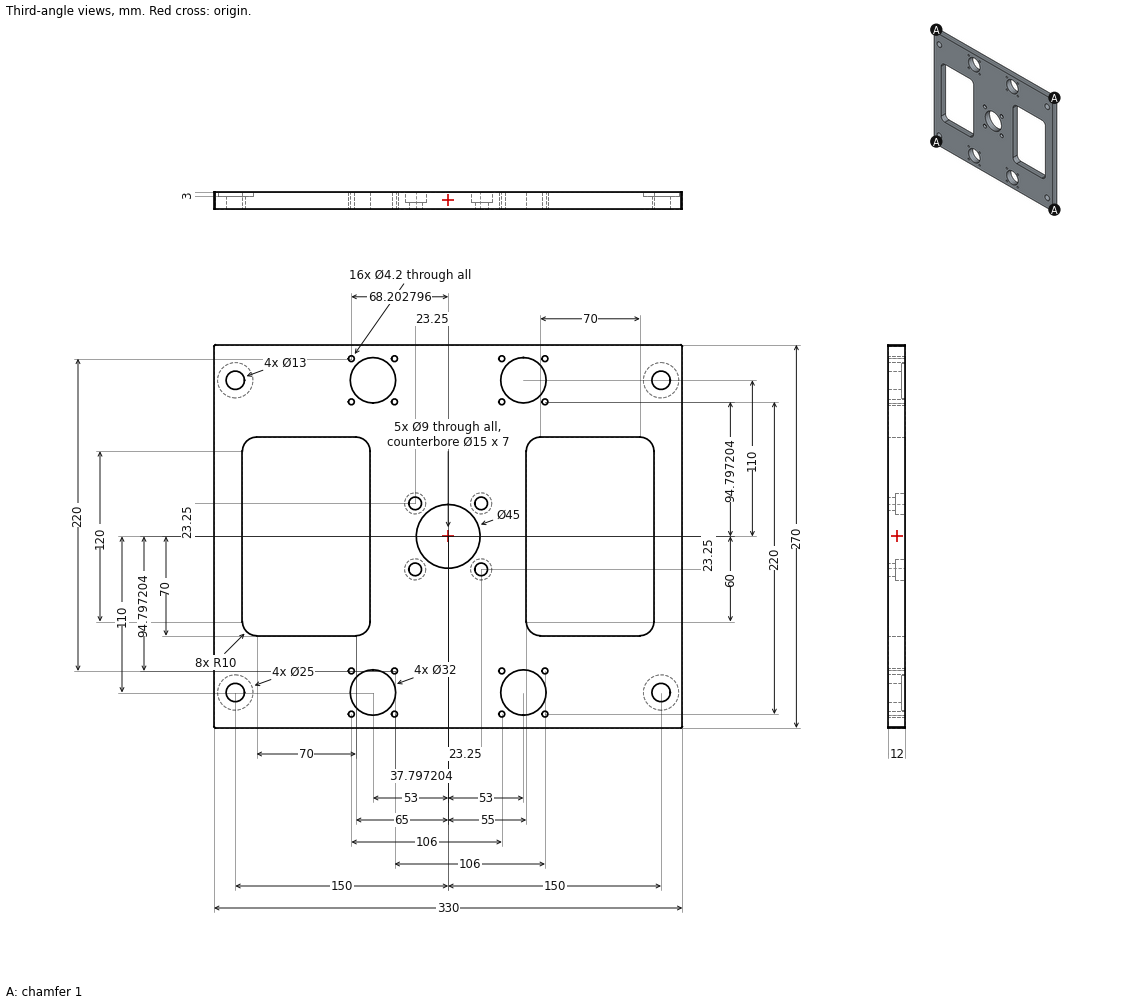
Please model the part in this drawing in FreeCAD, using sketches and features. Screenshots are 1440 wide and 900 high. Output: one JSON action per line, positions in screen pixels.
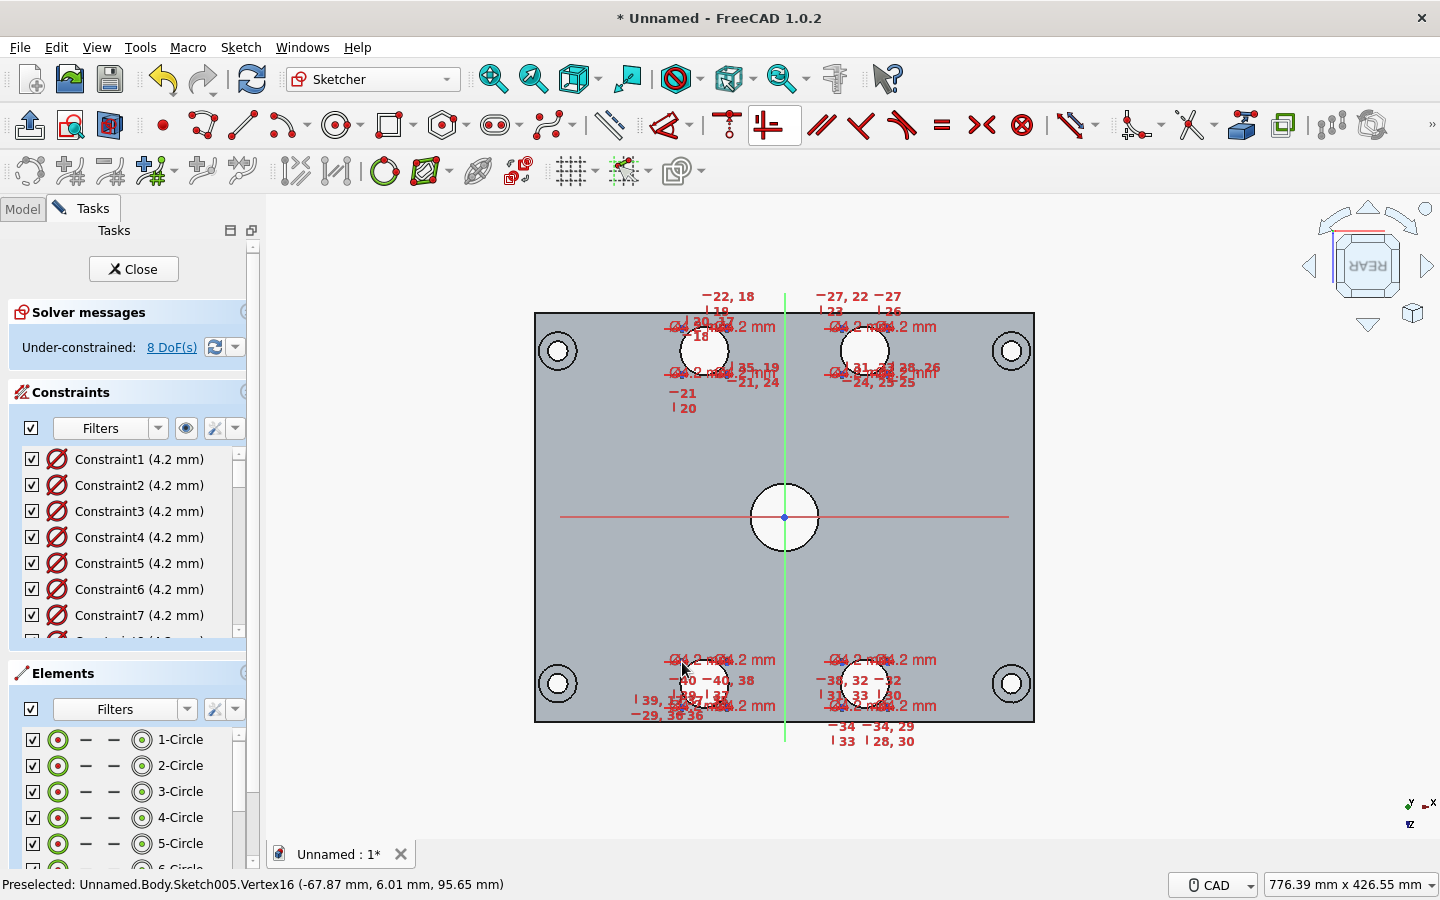
{"action": "left_click", "coordinate": [664, 126]}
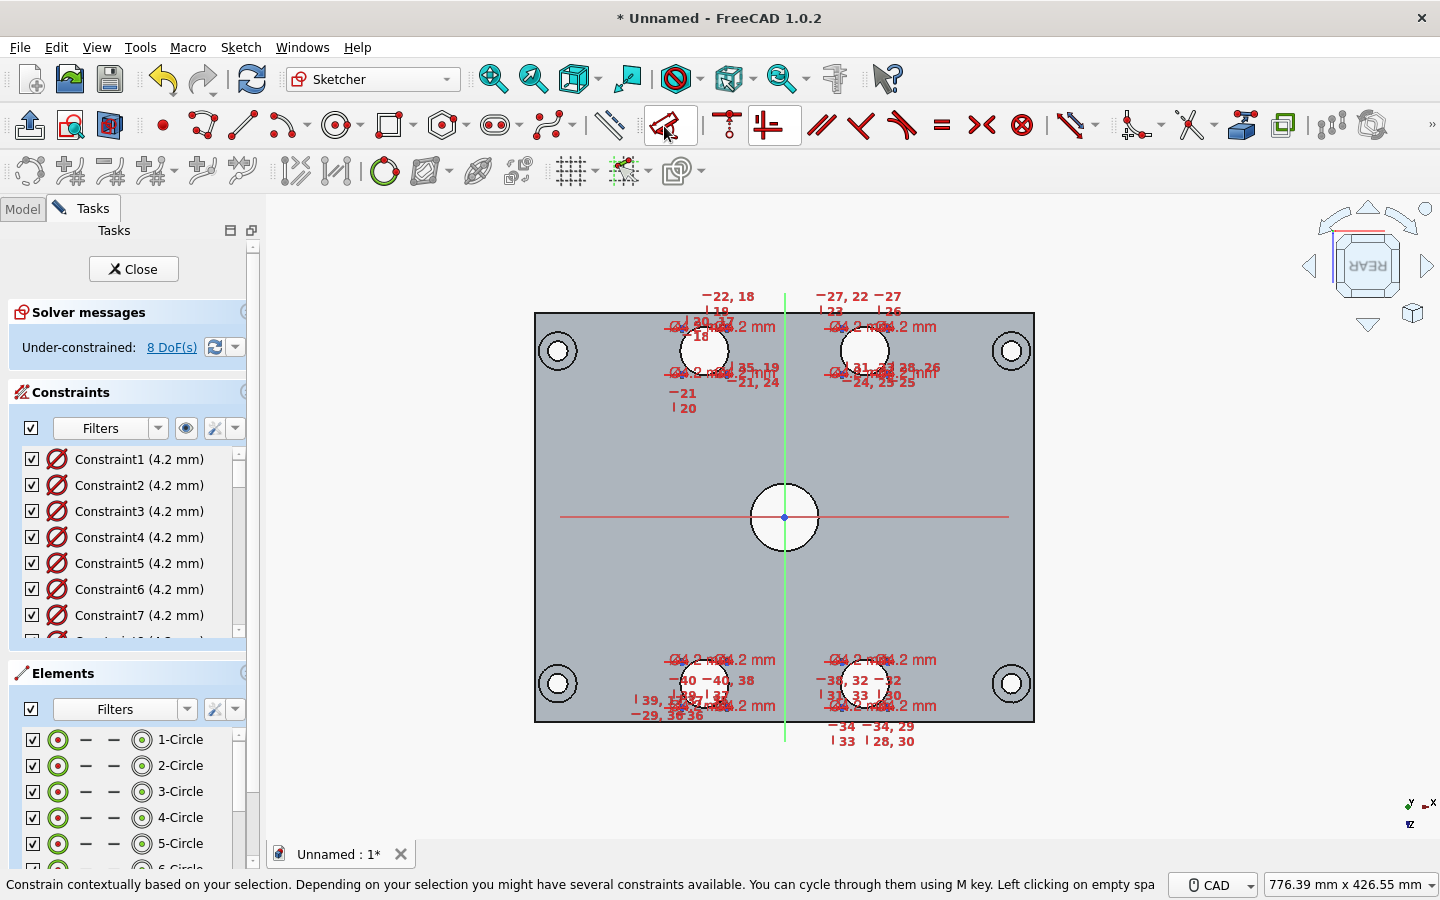
{"action": "left_click", "coordinate": [682, 708]}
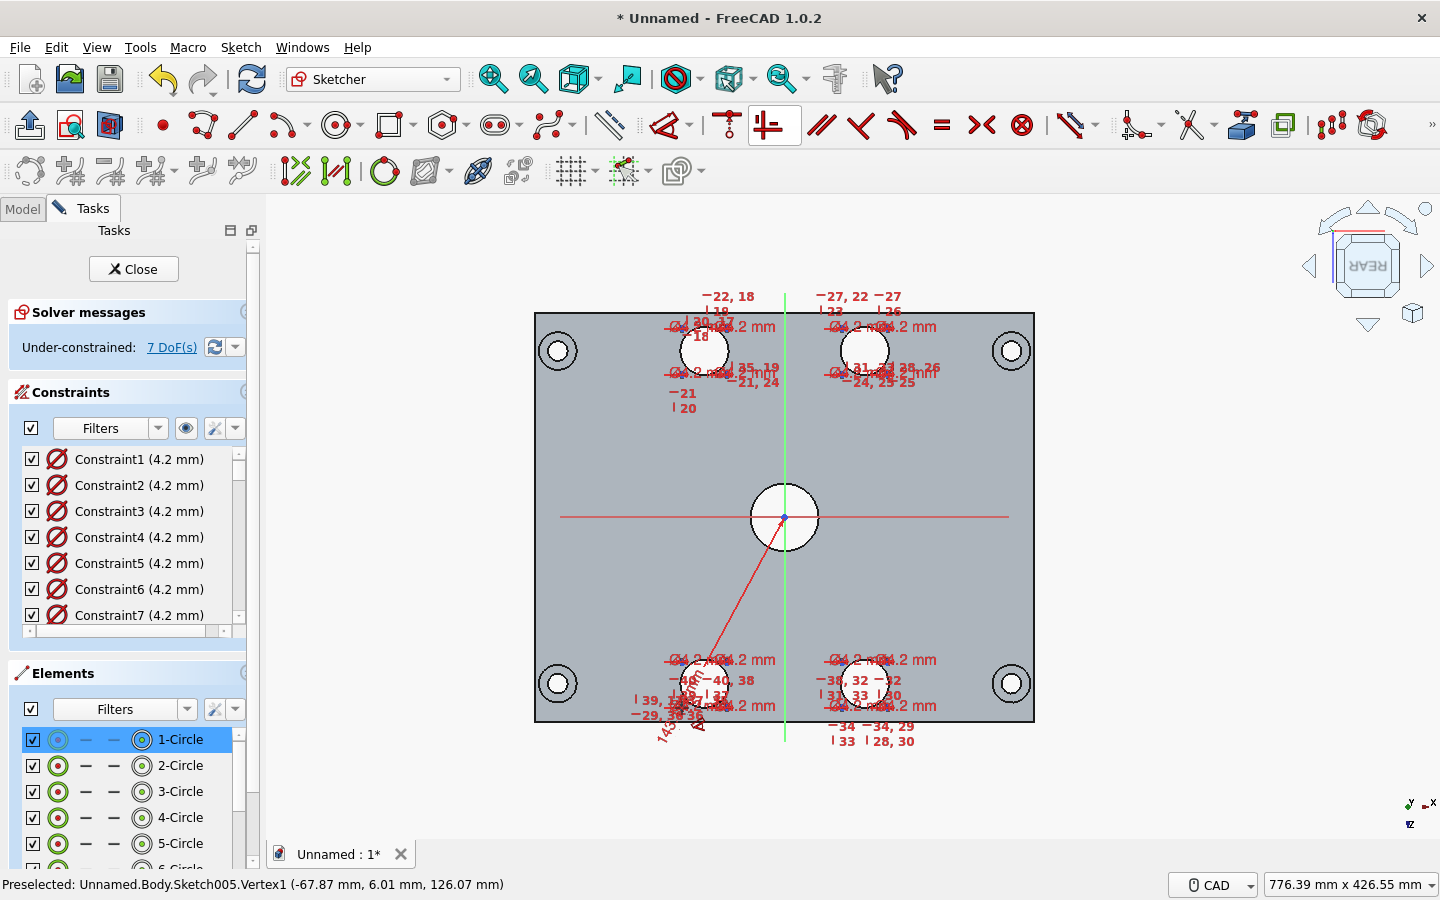
{"action": "left_click", "coordinate": [727, 375]}
{"action": "left_click", "coordinate": [648, 541]}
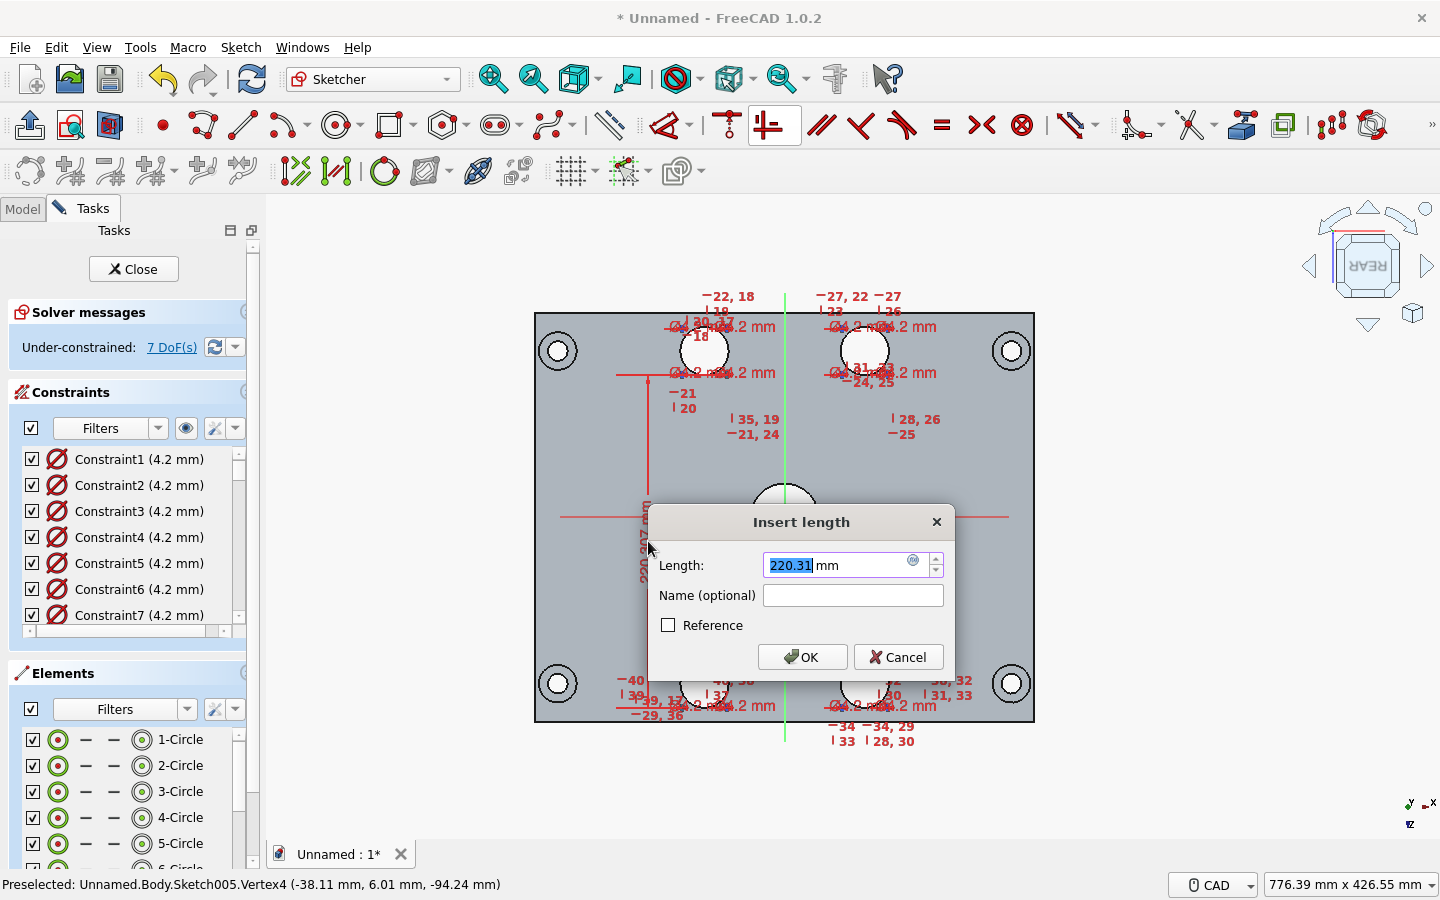
{"action": "type", "text": "220"}
{"action": "key", "text": "Return"}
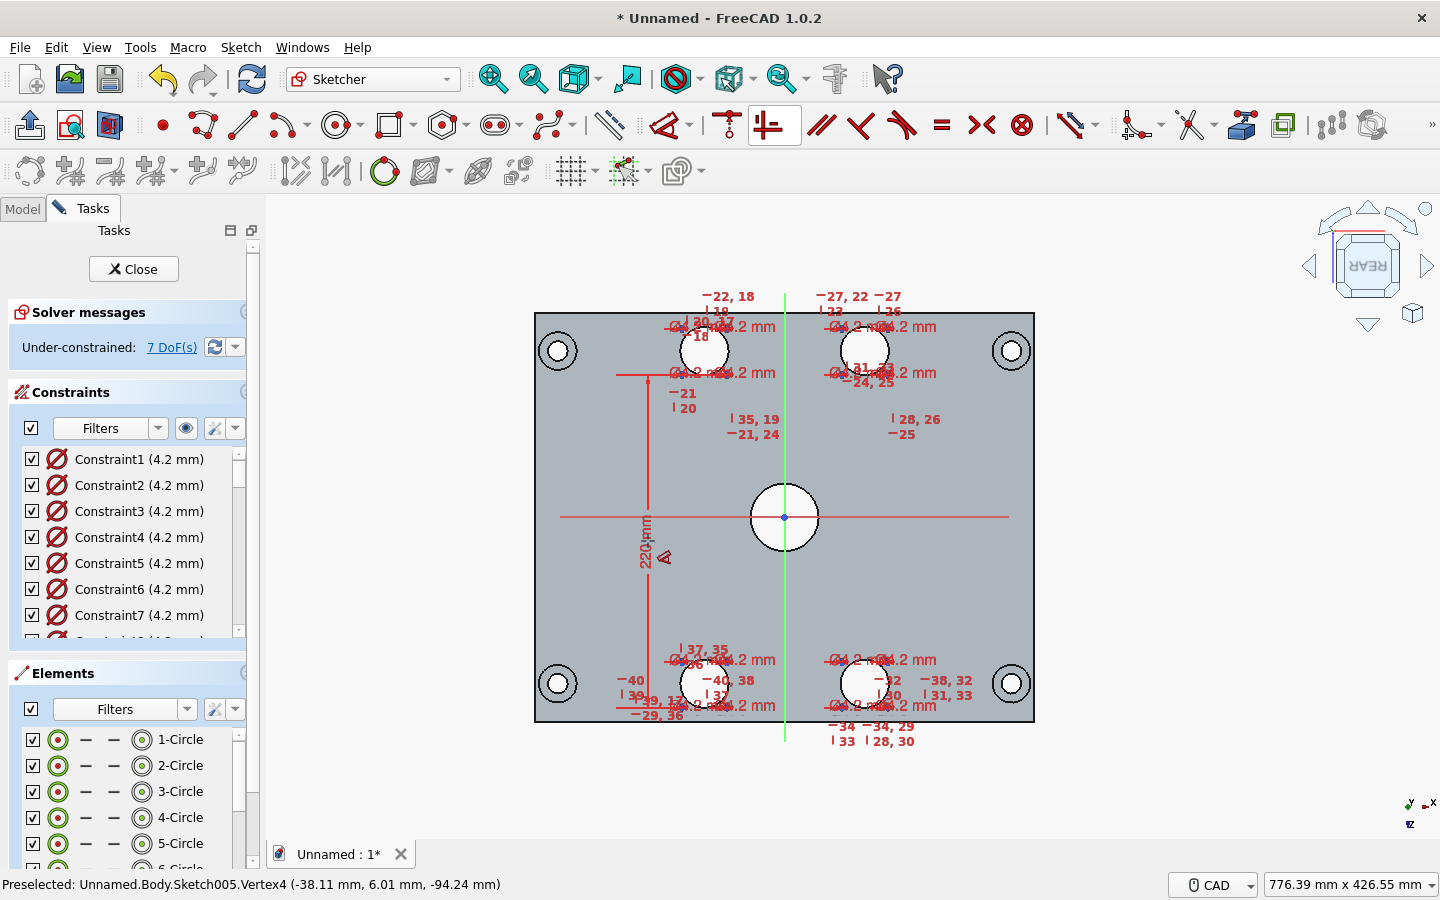
{"action": "left_click", "coordinate": [682, 329]}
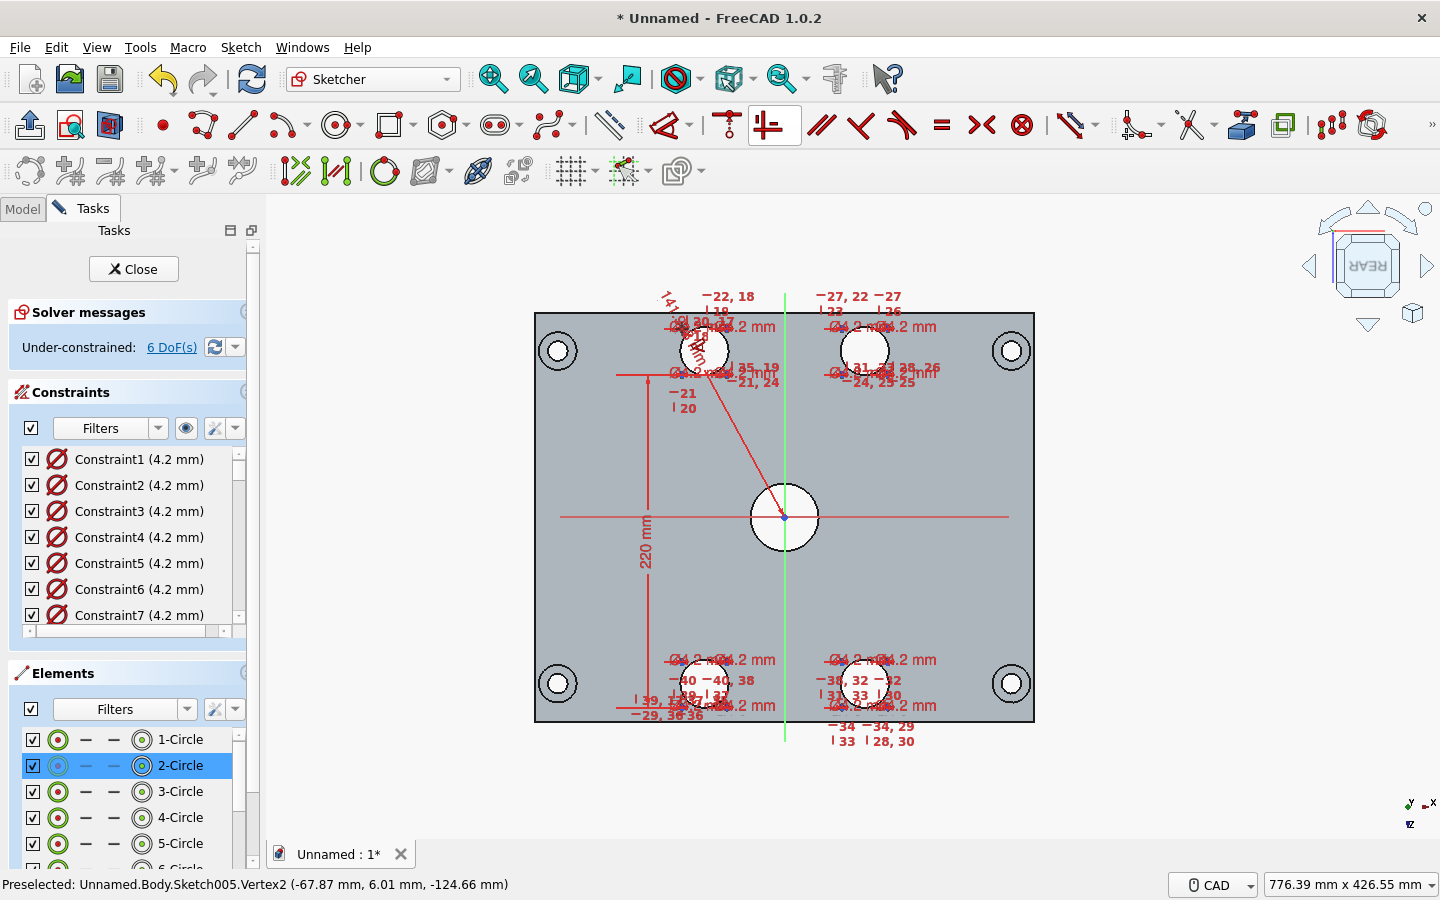
{"action": "left_click", "coordinate": [842, 329]}
{"action": "left_click", "coordinate": [762, 295]}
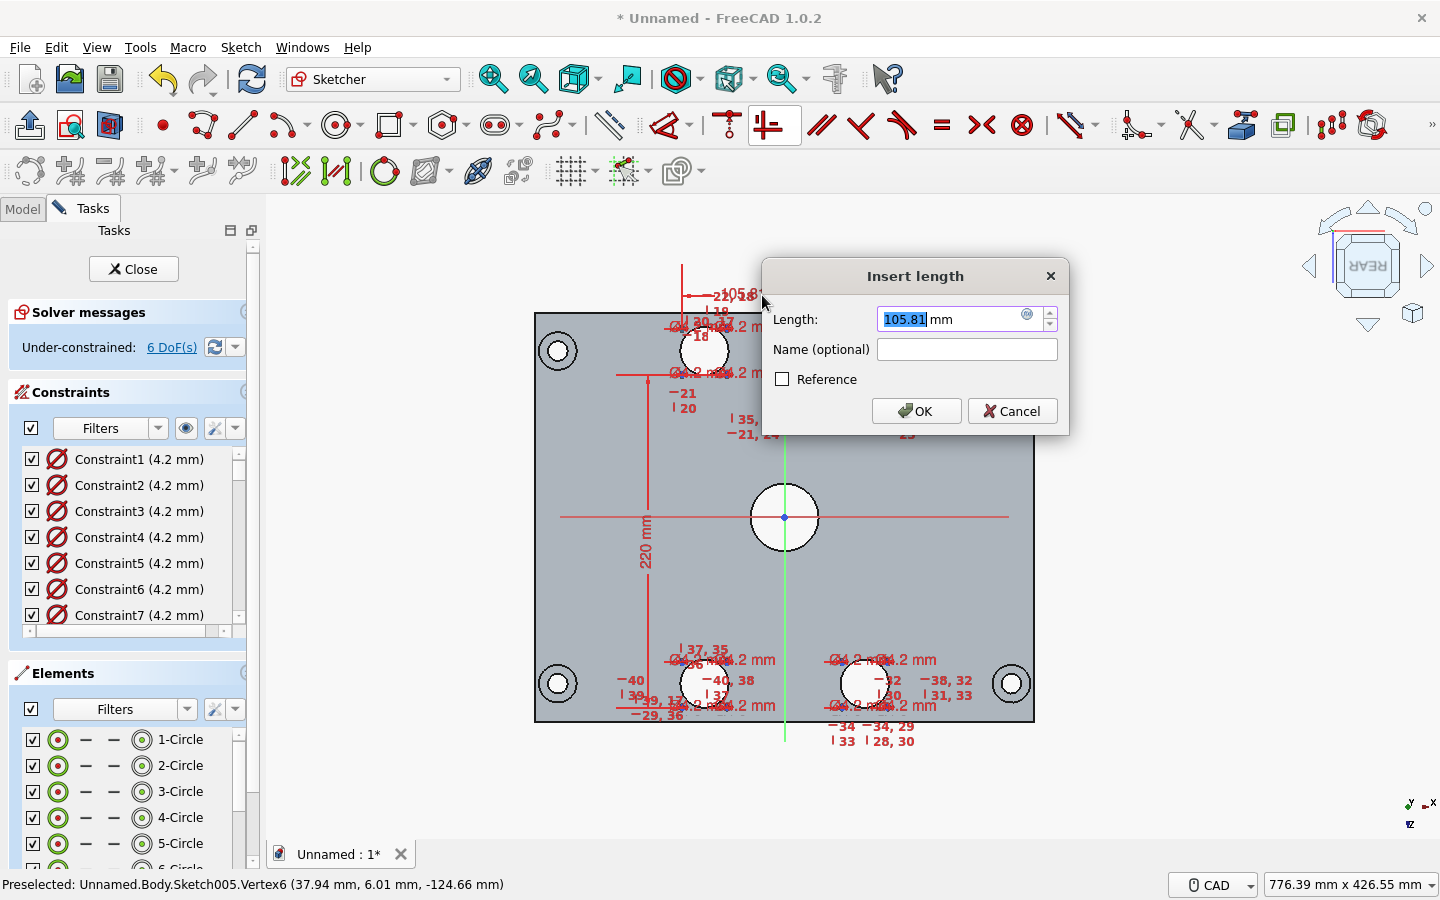
{"action": "type", "text": "106"}
{"action": "key", "text": "Return"}